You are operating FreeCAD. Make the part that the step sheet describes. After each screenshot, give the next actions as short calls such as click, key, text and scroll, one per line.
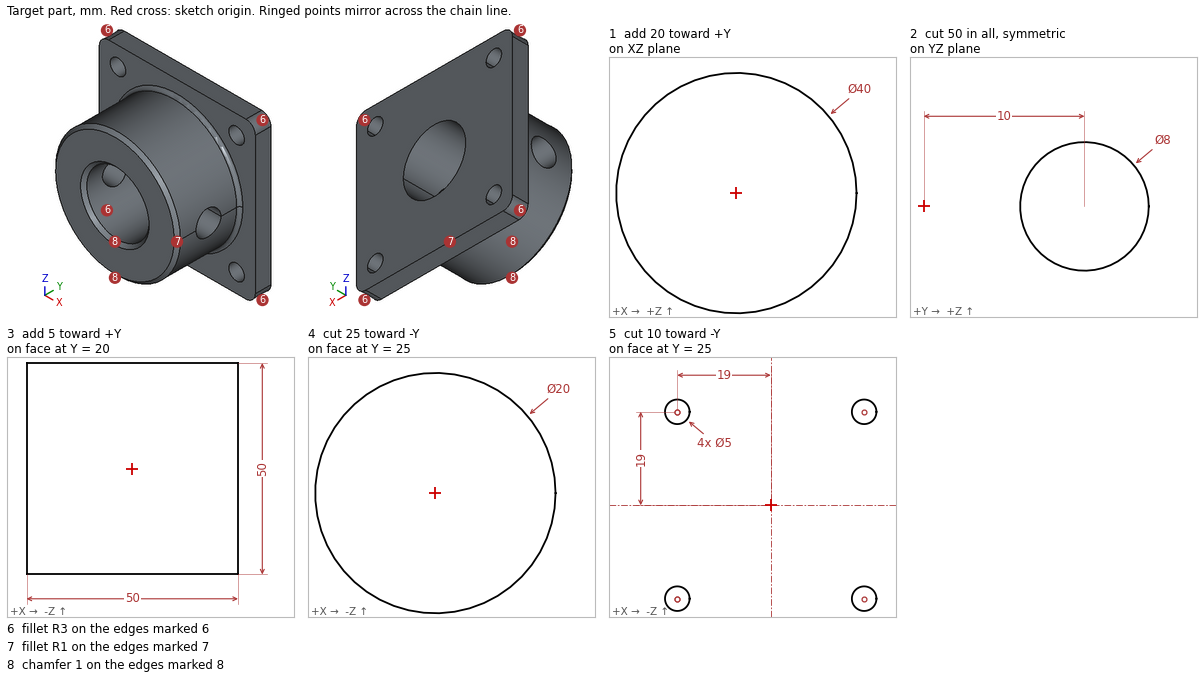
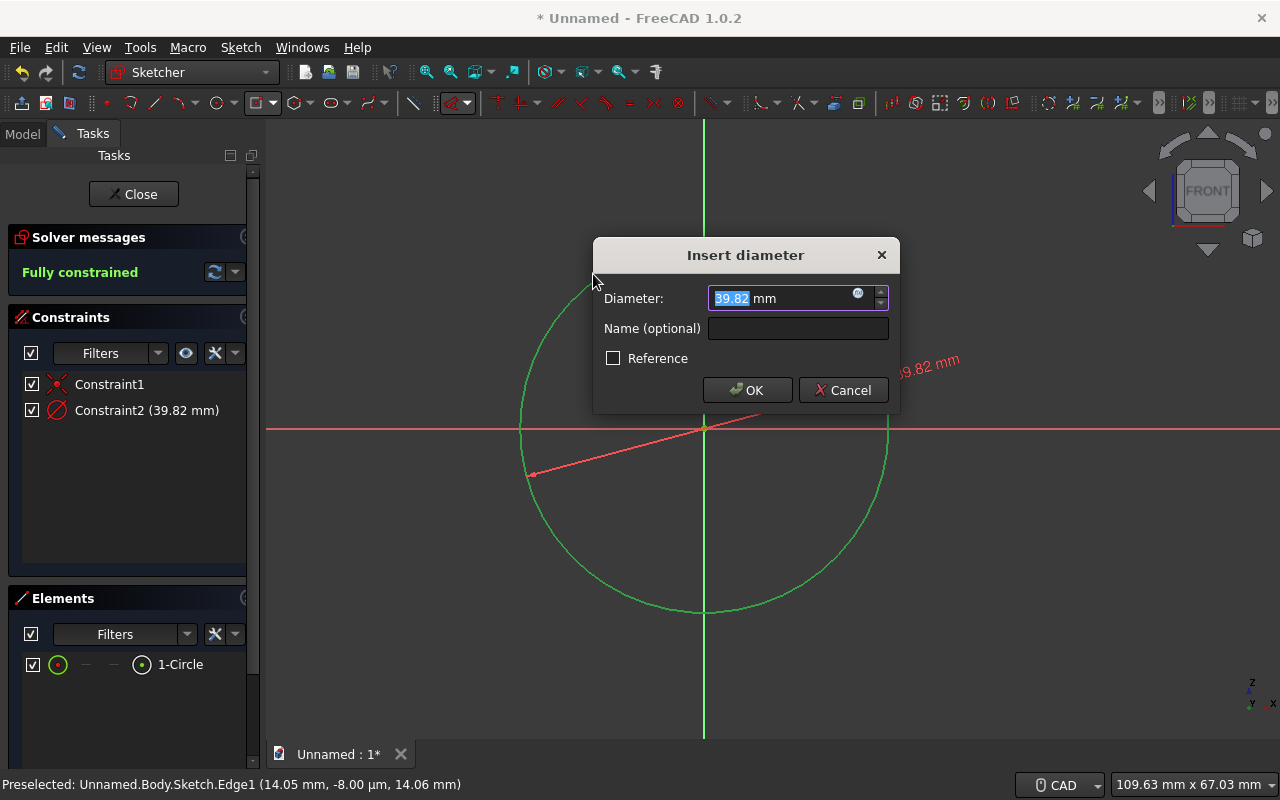
text(40)
key(Return)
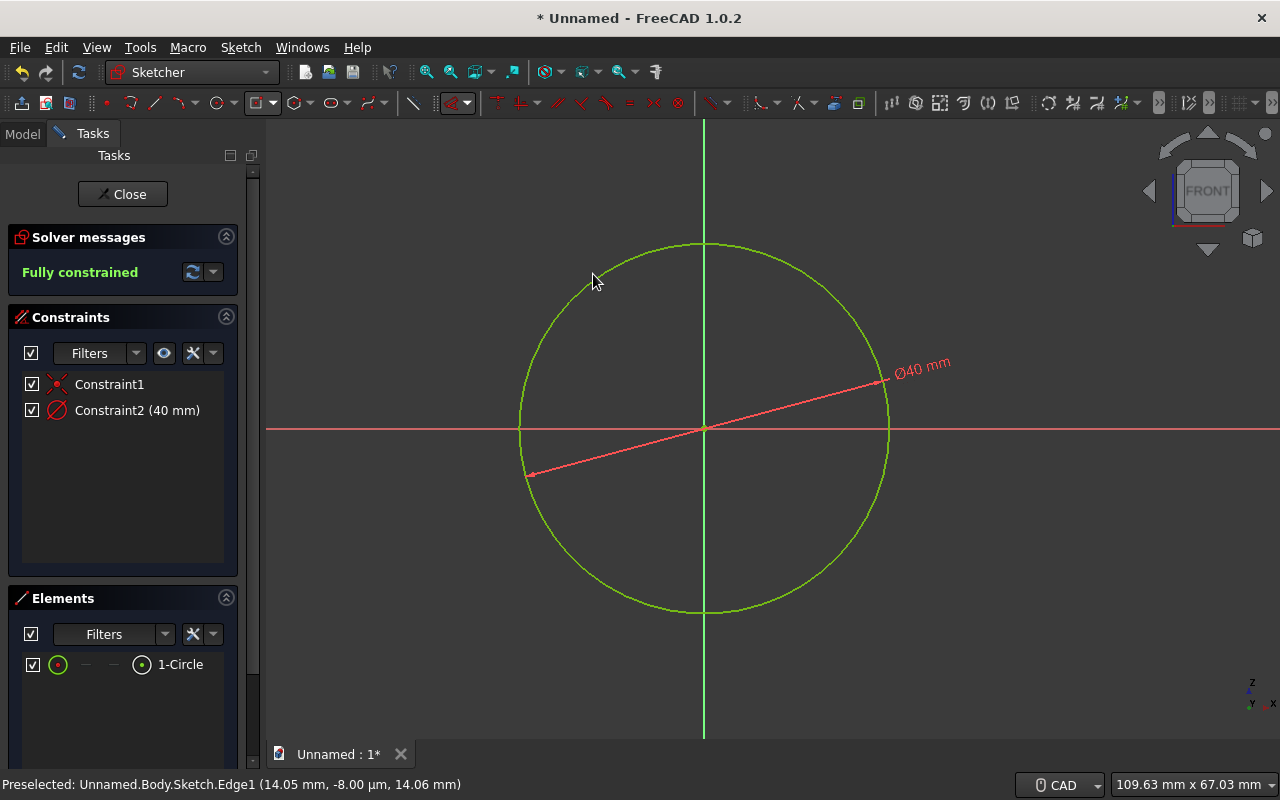
click(123, 194)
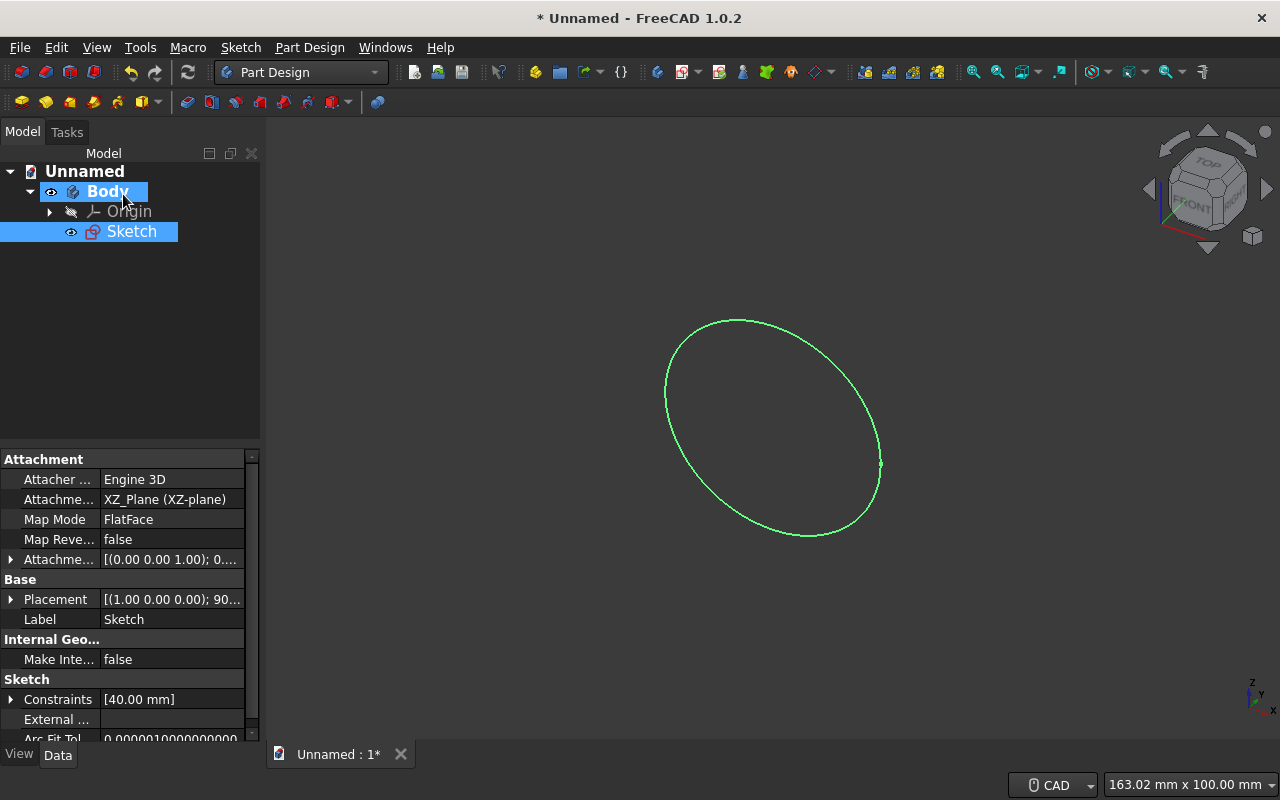
click(22, 102)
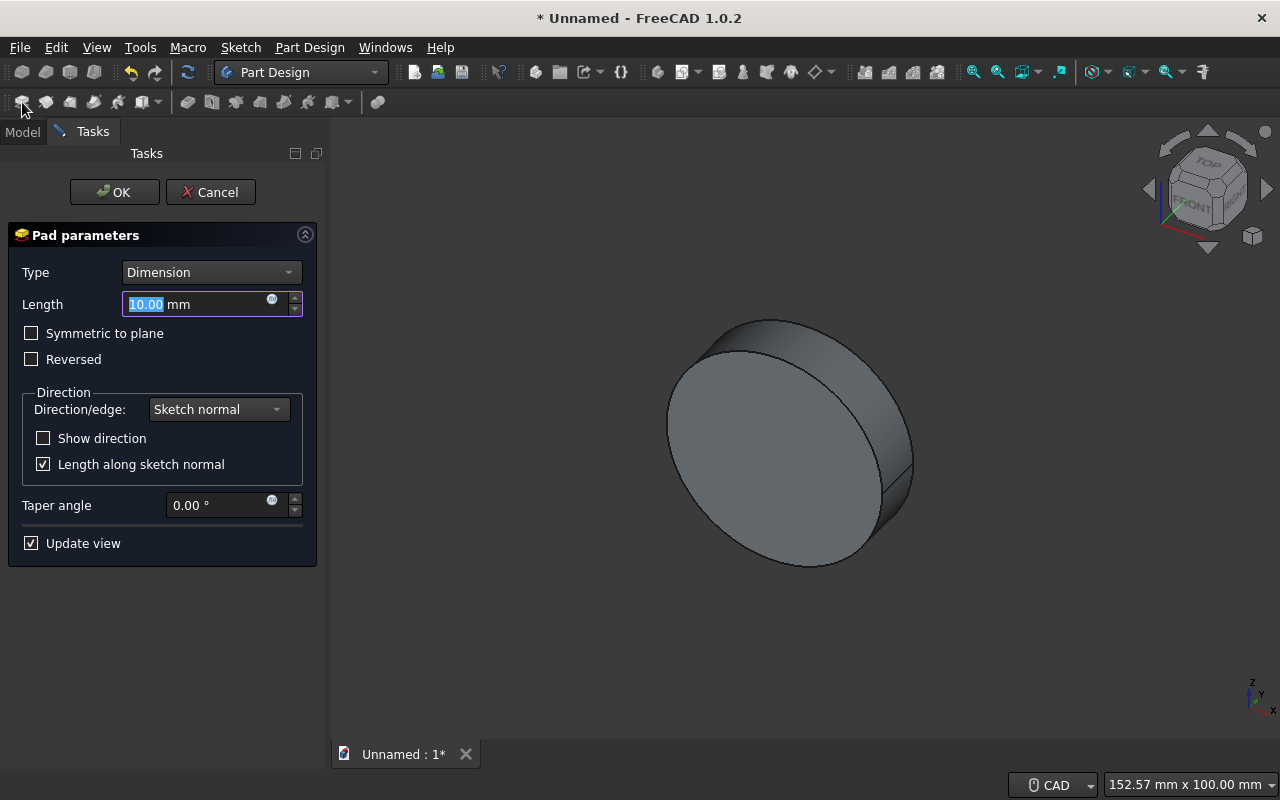
text(20)
key(Tab)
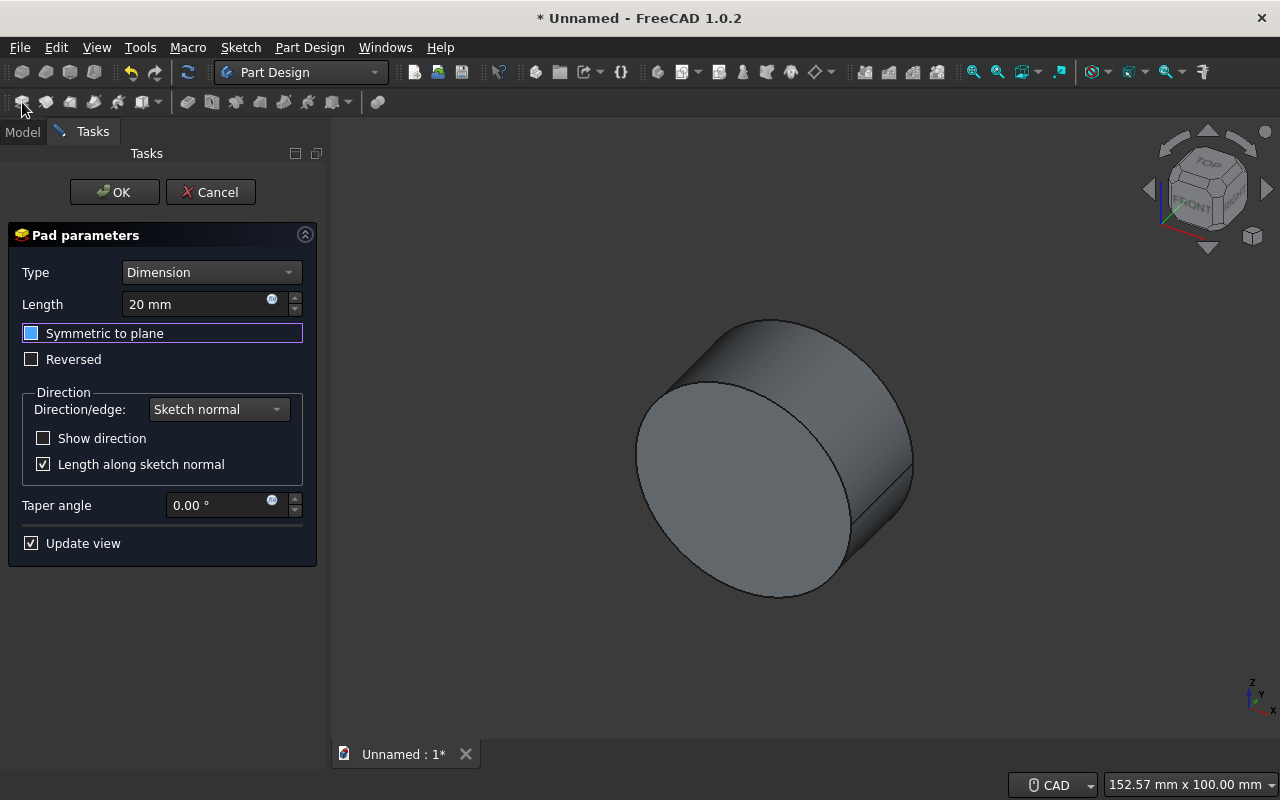
click(30, 359)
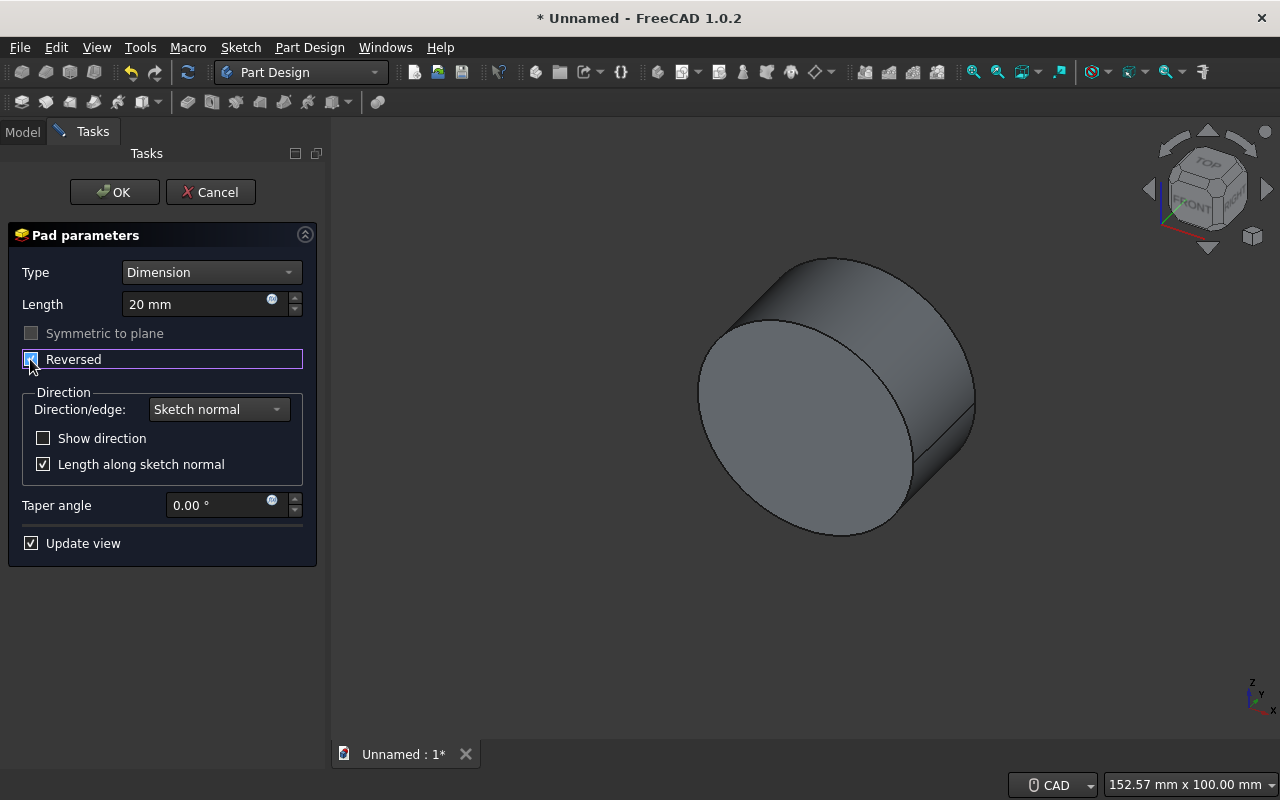
click(115, 192)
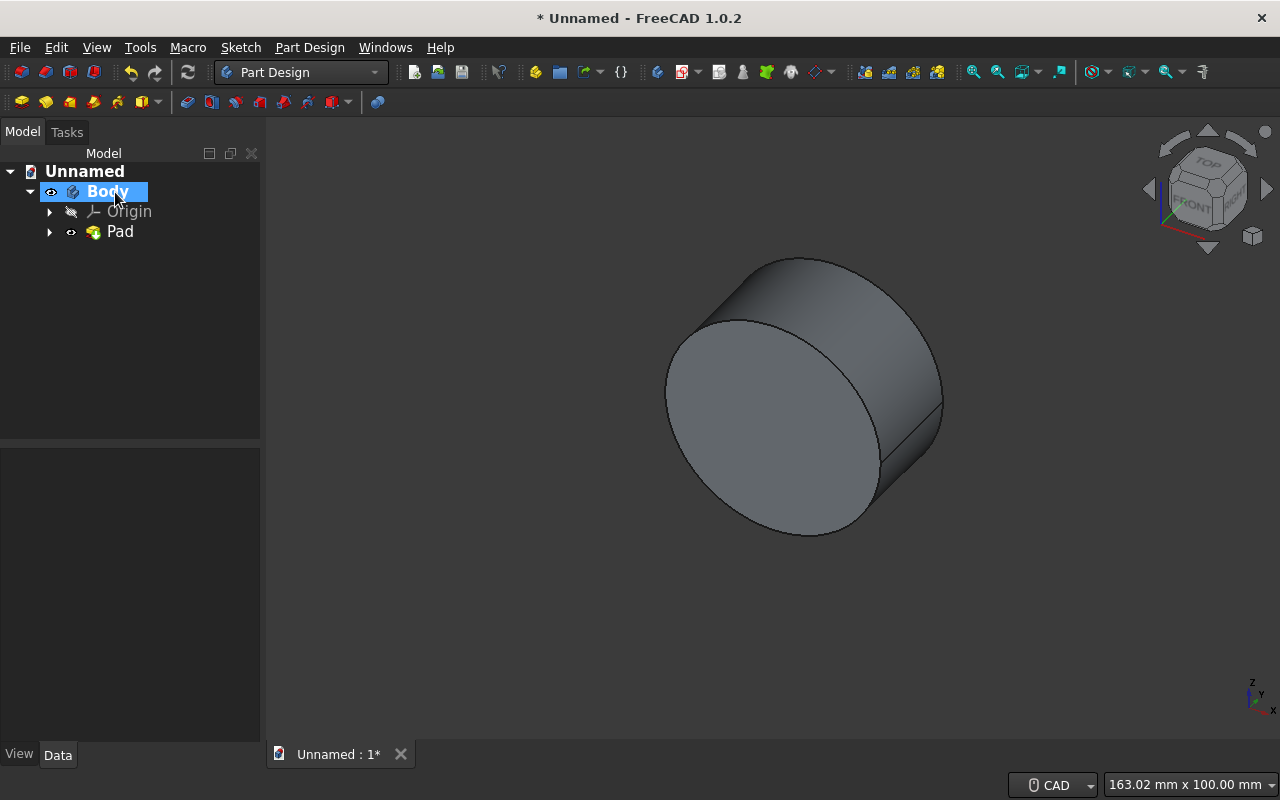
click(682, 72)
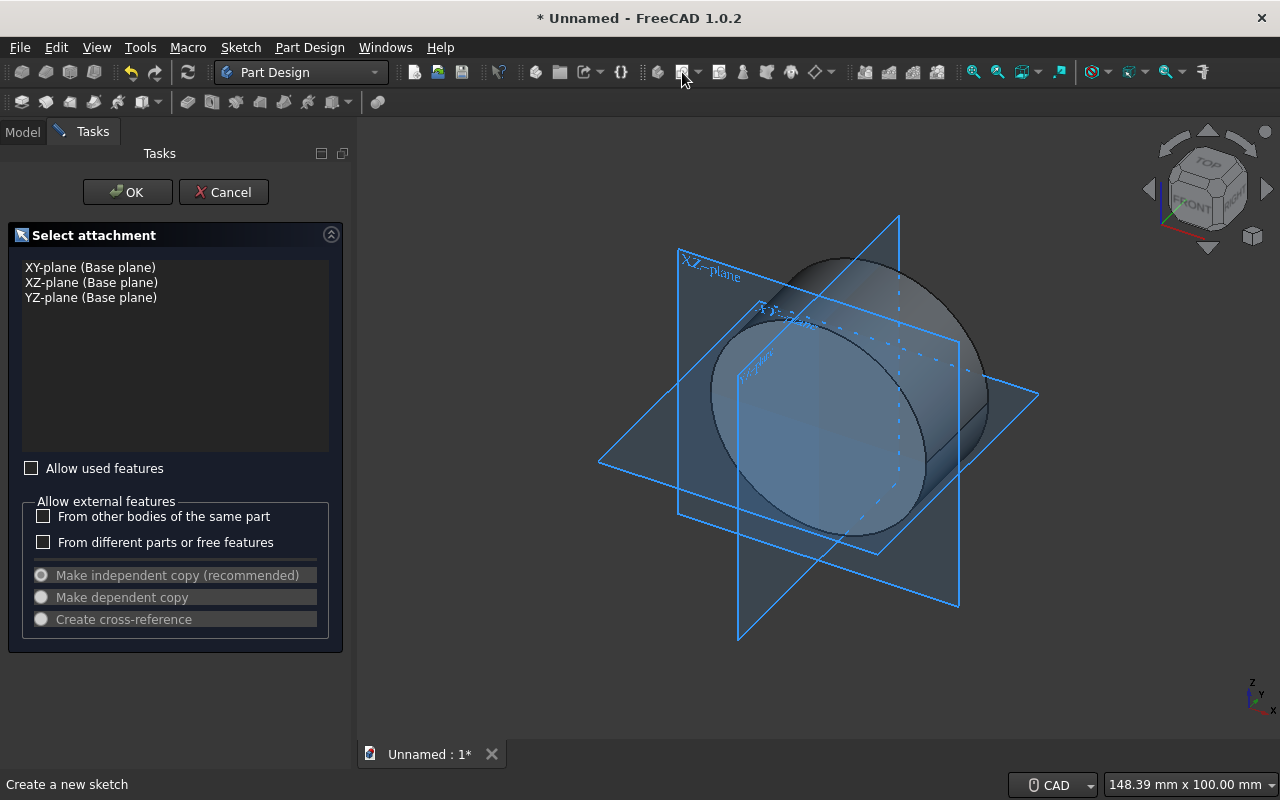
click(82, 298)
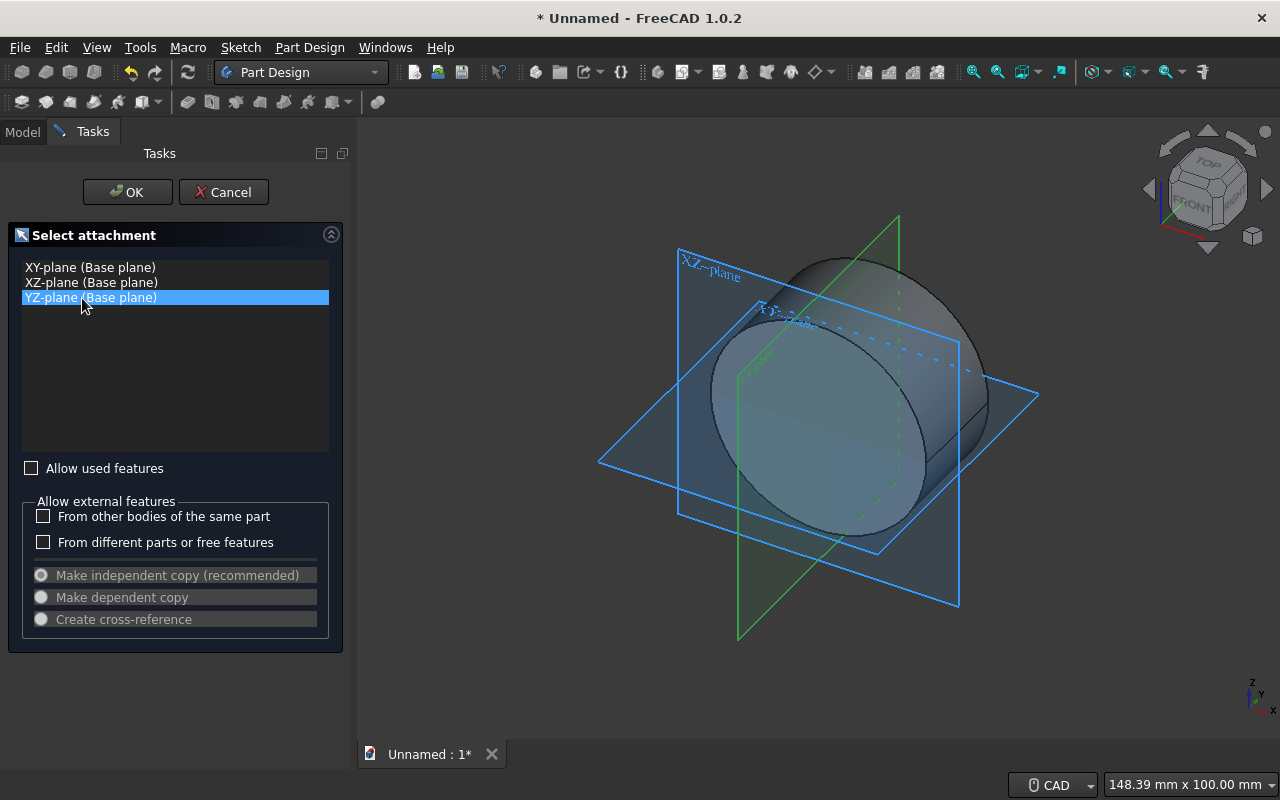
click(128, 192)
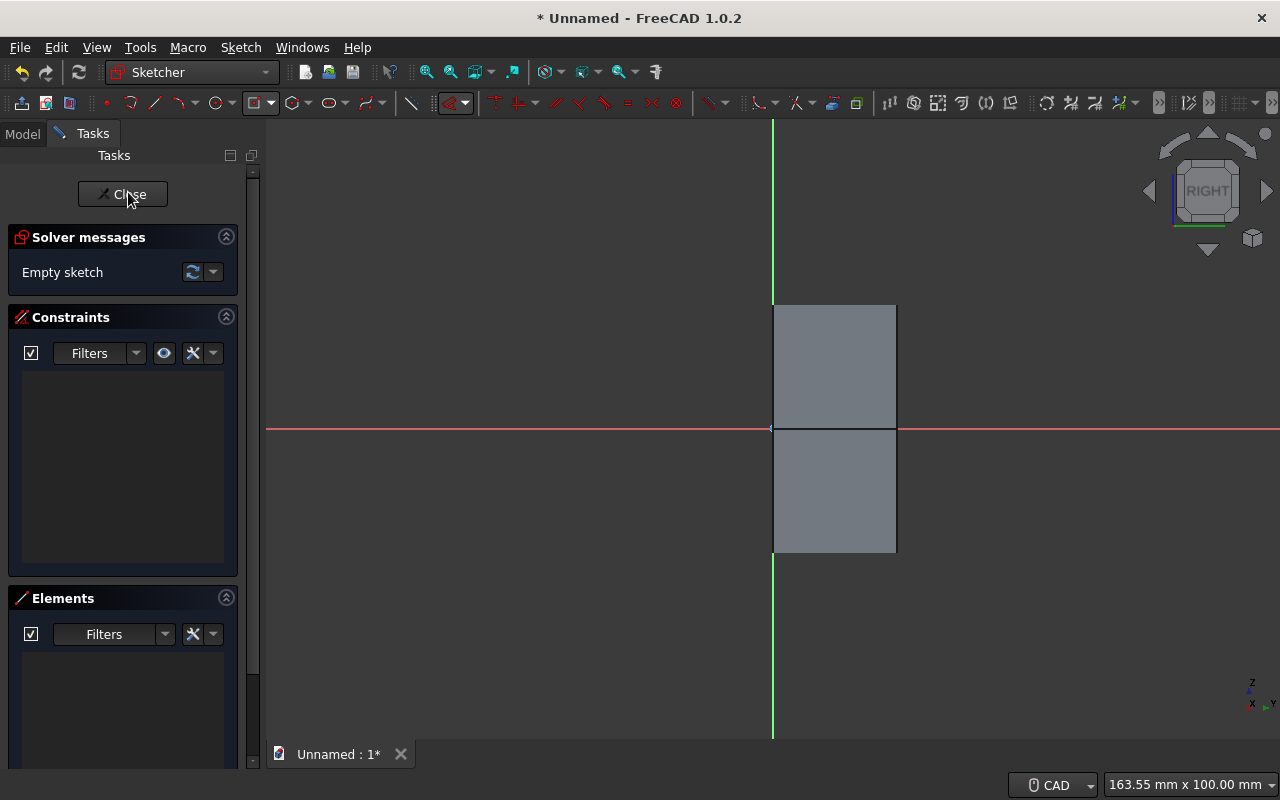
click(70, 104)